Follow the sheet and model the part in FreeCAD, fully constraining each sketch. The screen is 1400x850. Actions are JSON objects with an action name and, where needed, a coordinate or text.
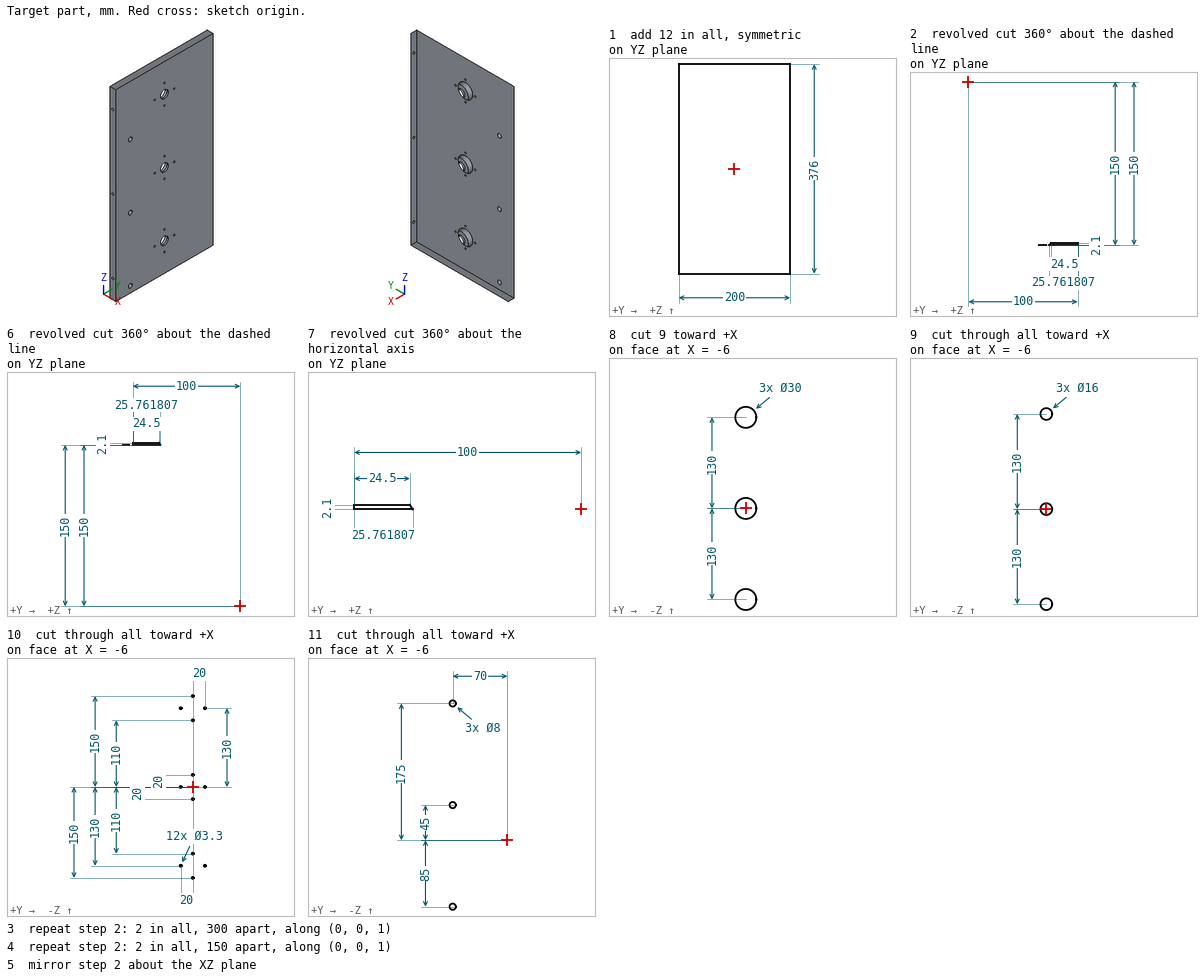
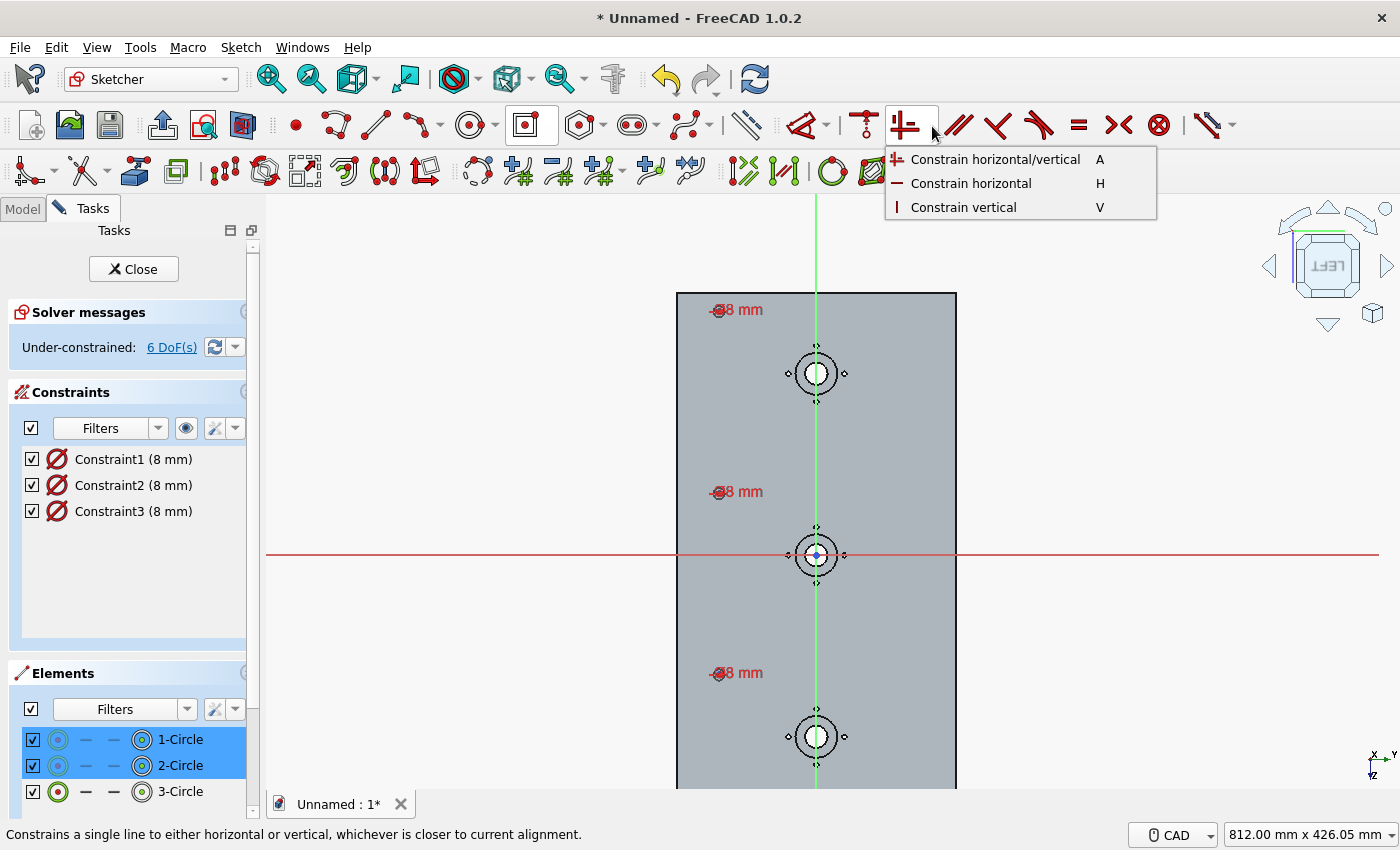
{"action": "left_click", "coordinate": [1021, 207]}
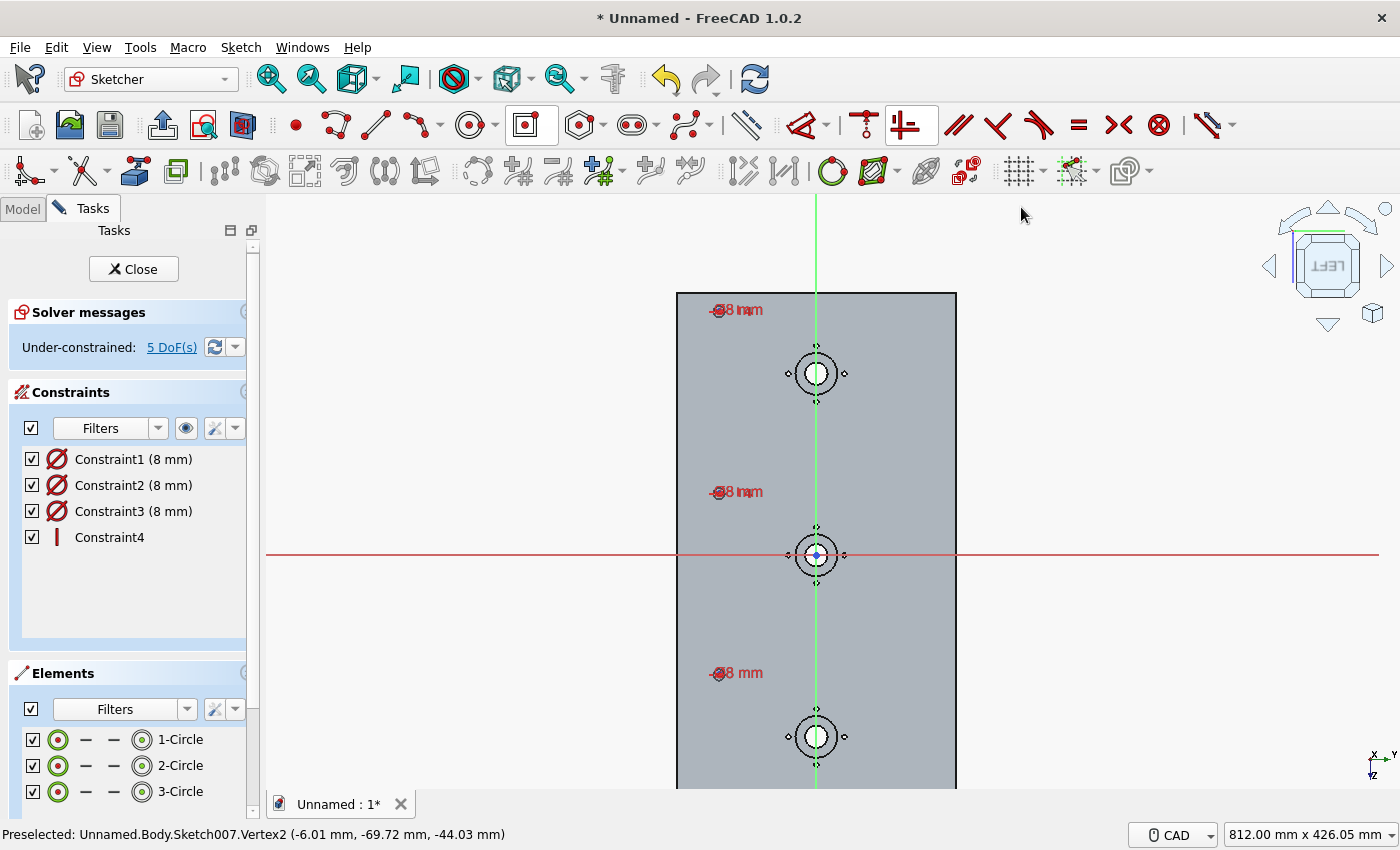
{"action": "left_click", "coordinate": [719, 494]}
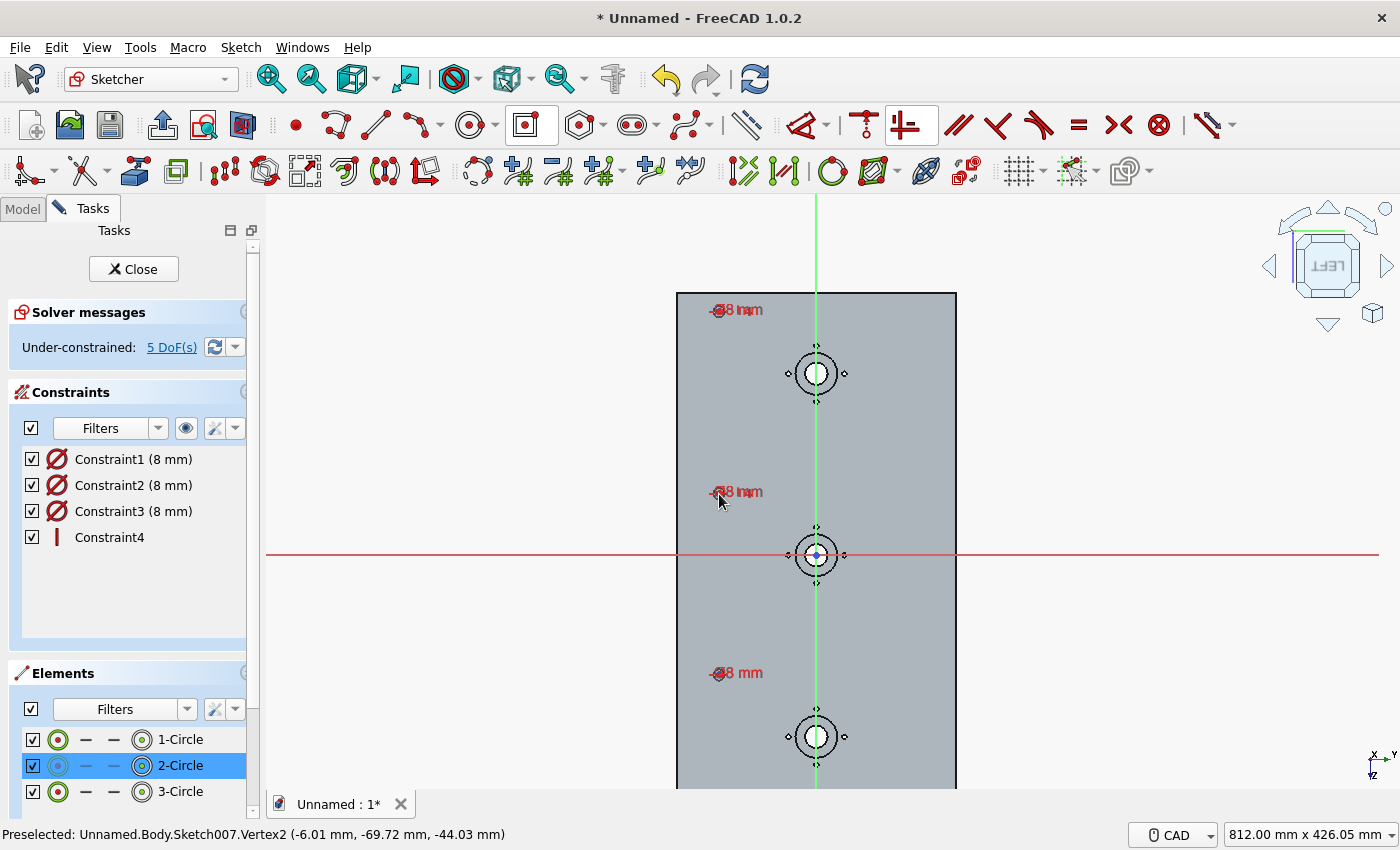
{"action": "left_click", "coordinate": [719, 675]}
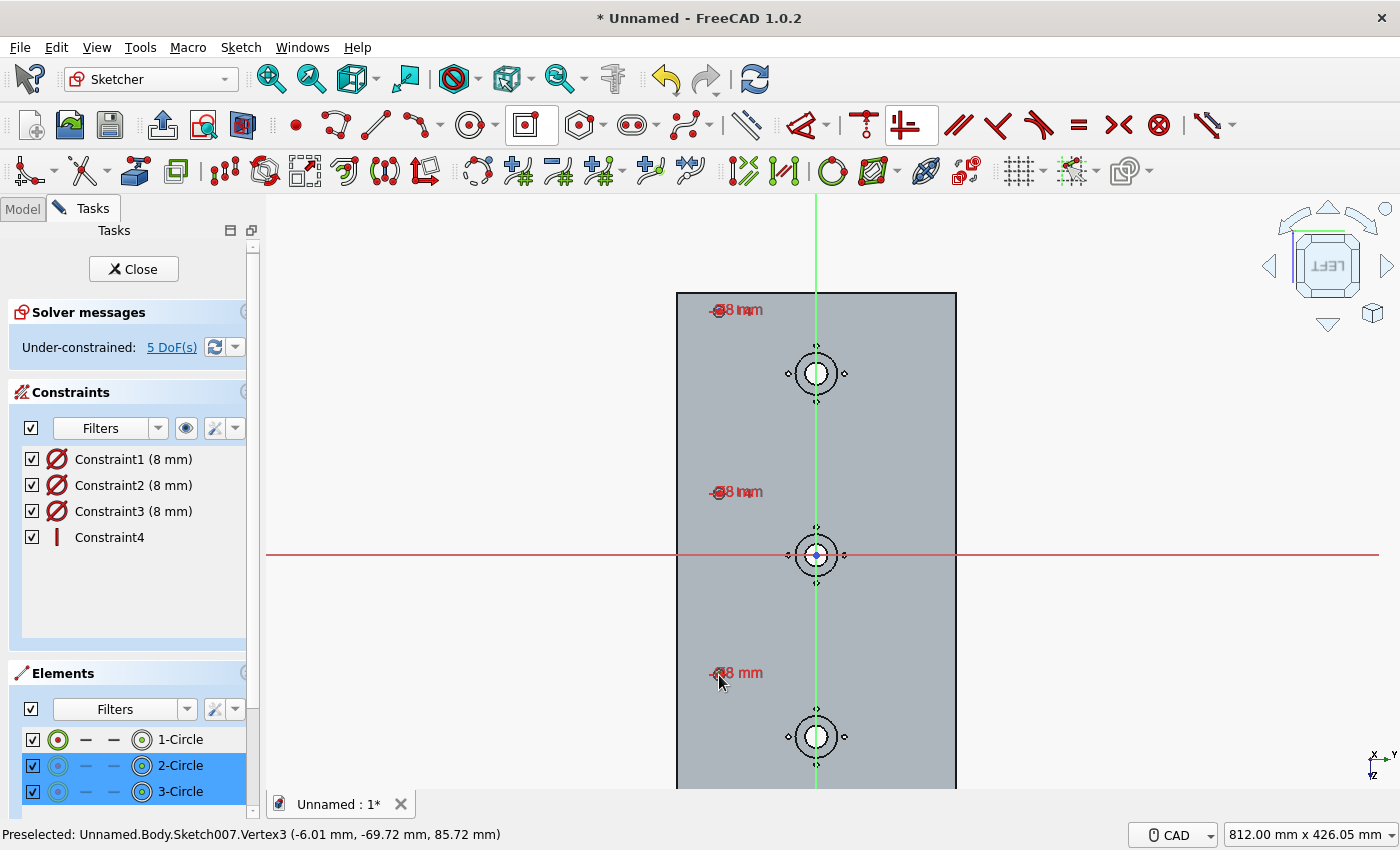
{"action": "left_click", "coordinate": [932, 126]}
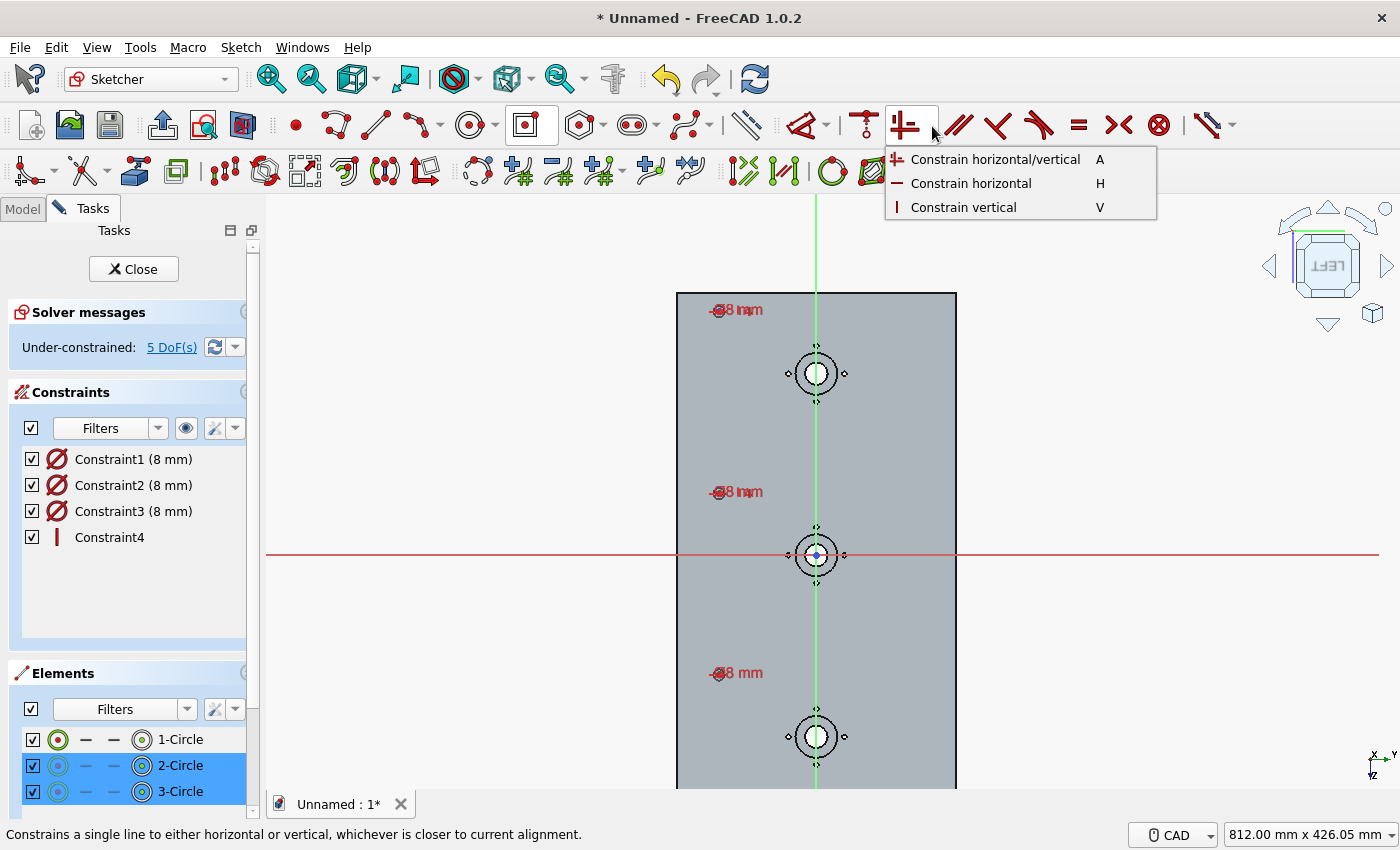
{"action": "left_click", "coordinate": [1021, 207]}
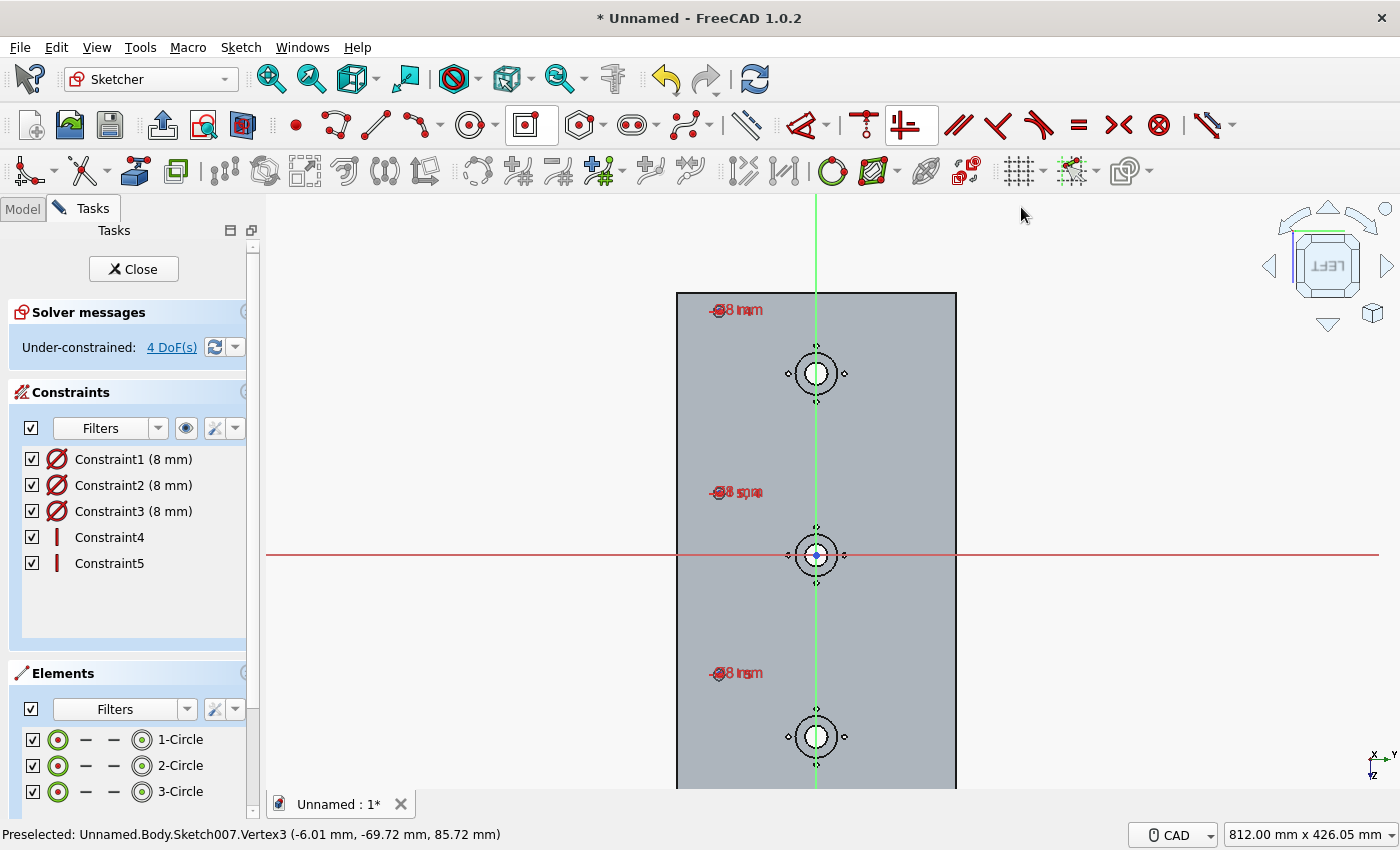
{"action": "left_click", "coordinate": [802, 126]}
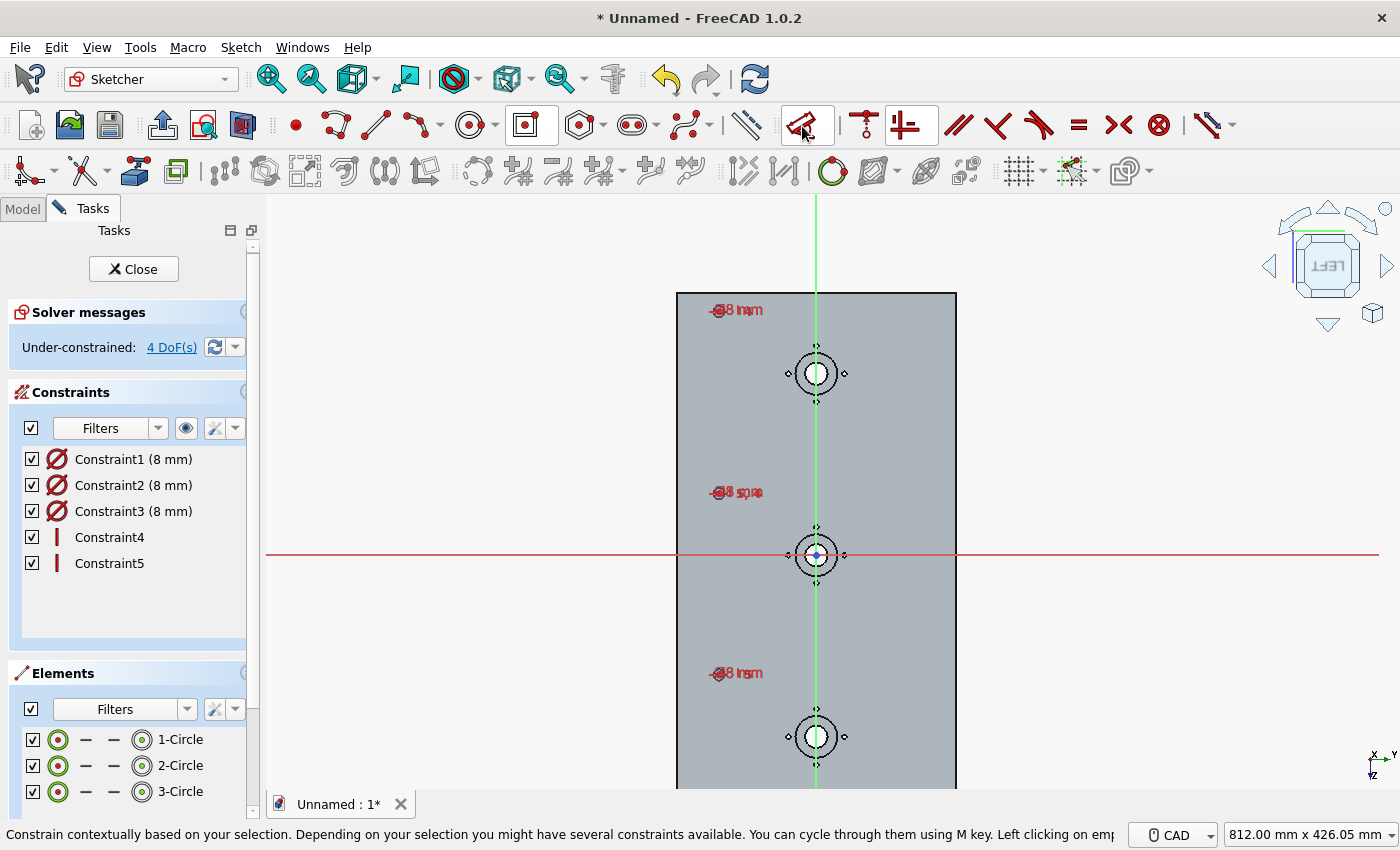
{"action": "left_click", "coordinate": [719, 312]}
{"action": "left_click", "coordinate": [768, 278]}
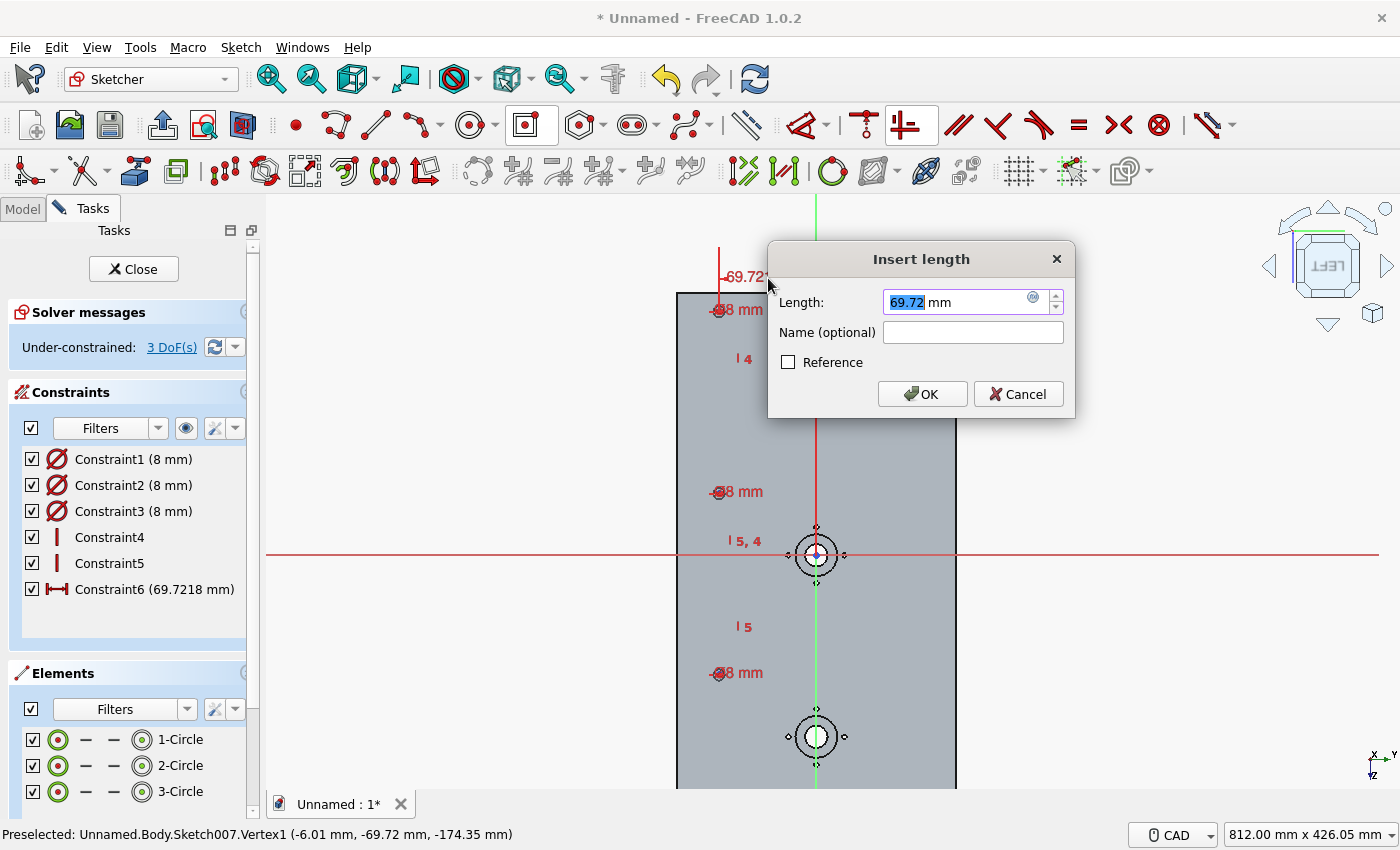
{"action": "type", "text": "70"}
{"action": "key", "text": "Return"}